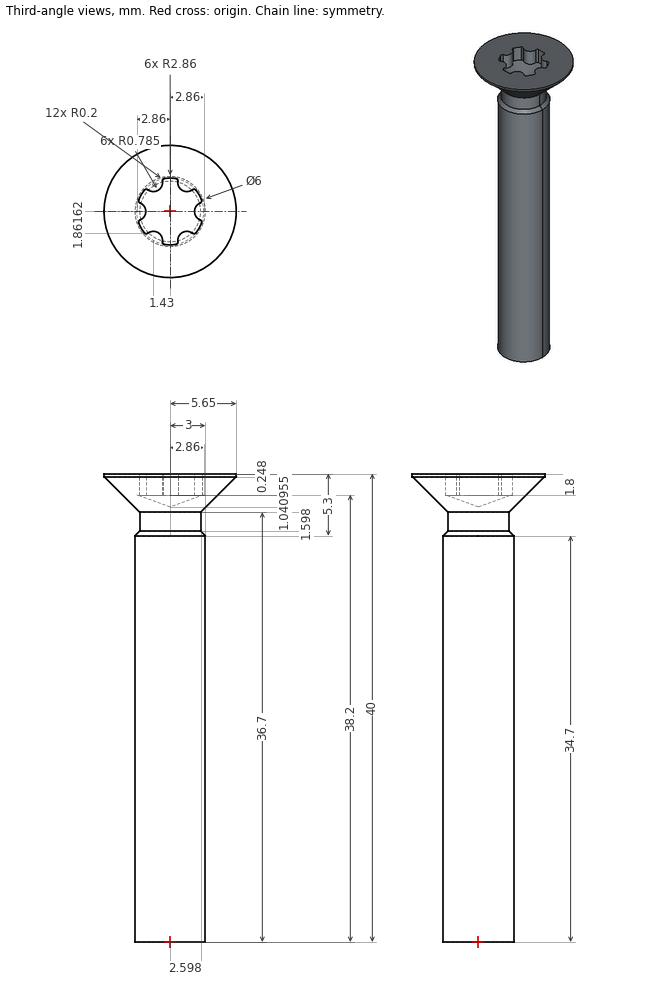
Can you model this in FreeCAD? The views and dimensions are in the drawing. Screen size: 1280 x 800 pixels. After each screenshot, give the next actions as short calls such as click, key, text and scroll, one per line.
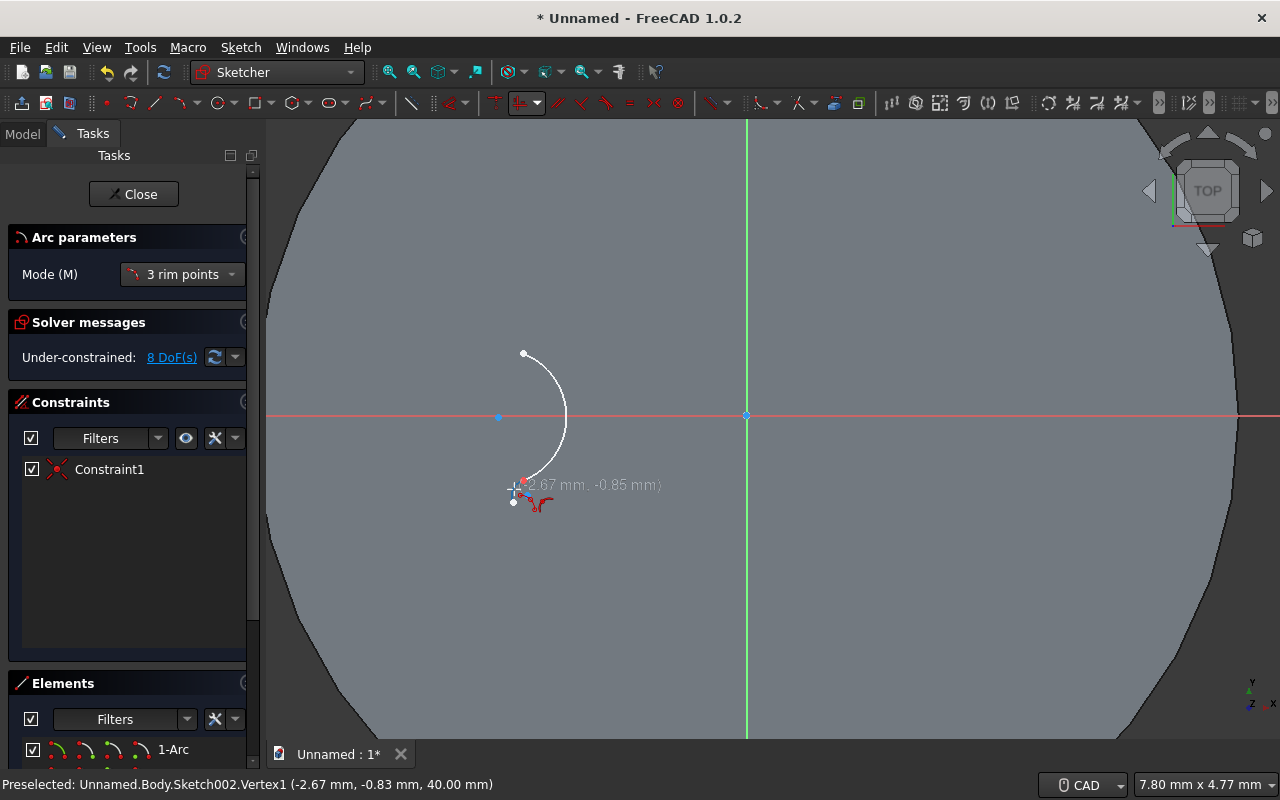
click(514, 500)
click(548, 560)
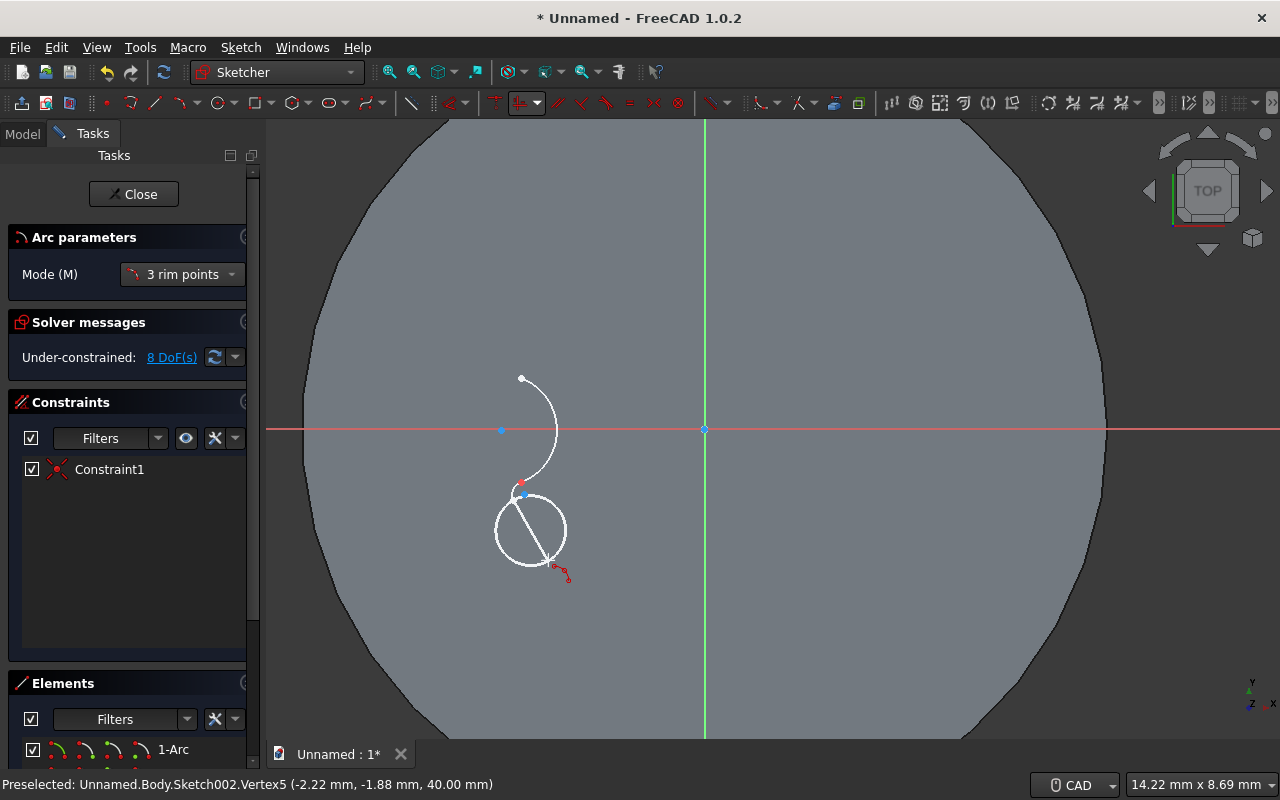
scroll(528, 531, up, 9)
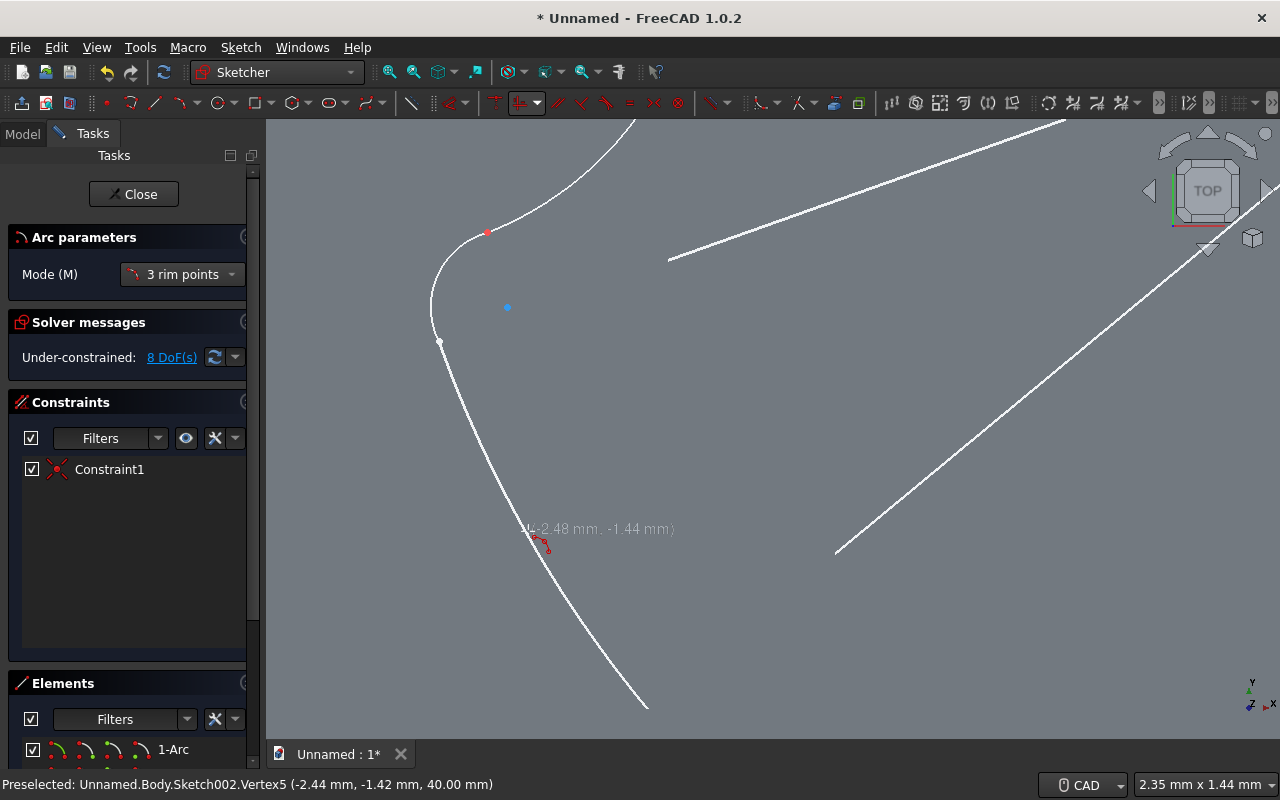
click(526, 529)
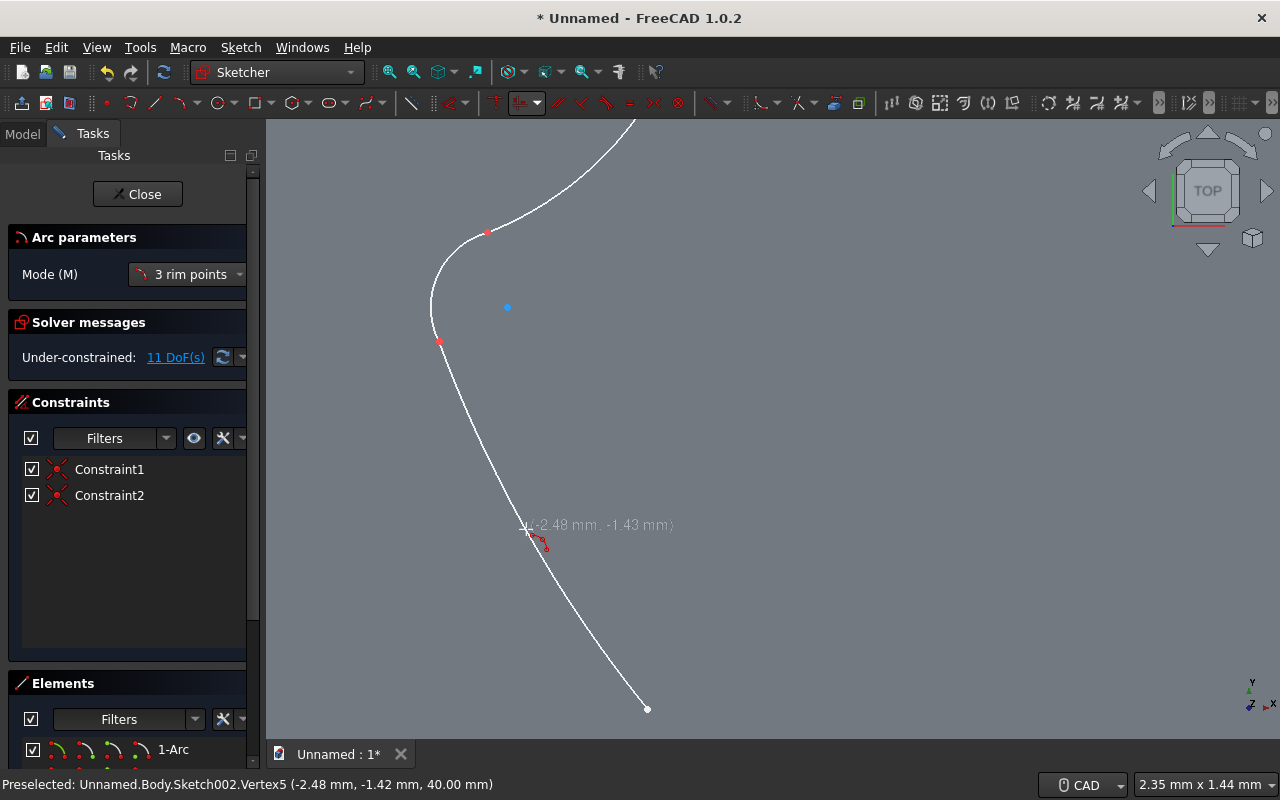
scroll(528, 531, down, 9)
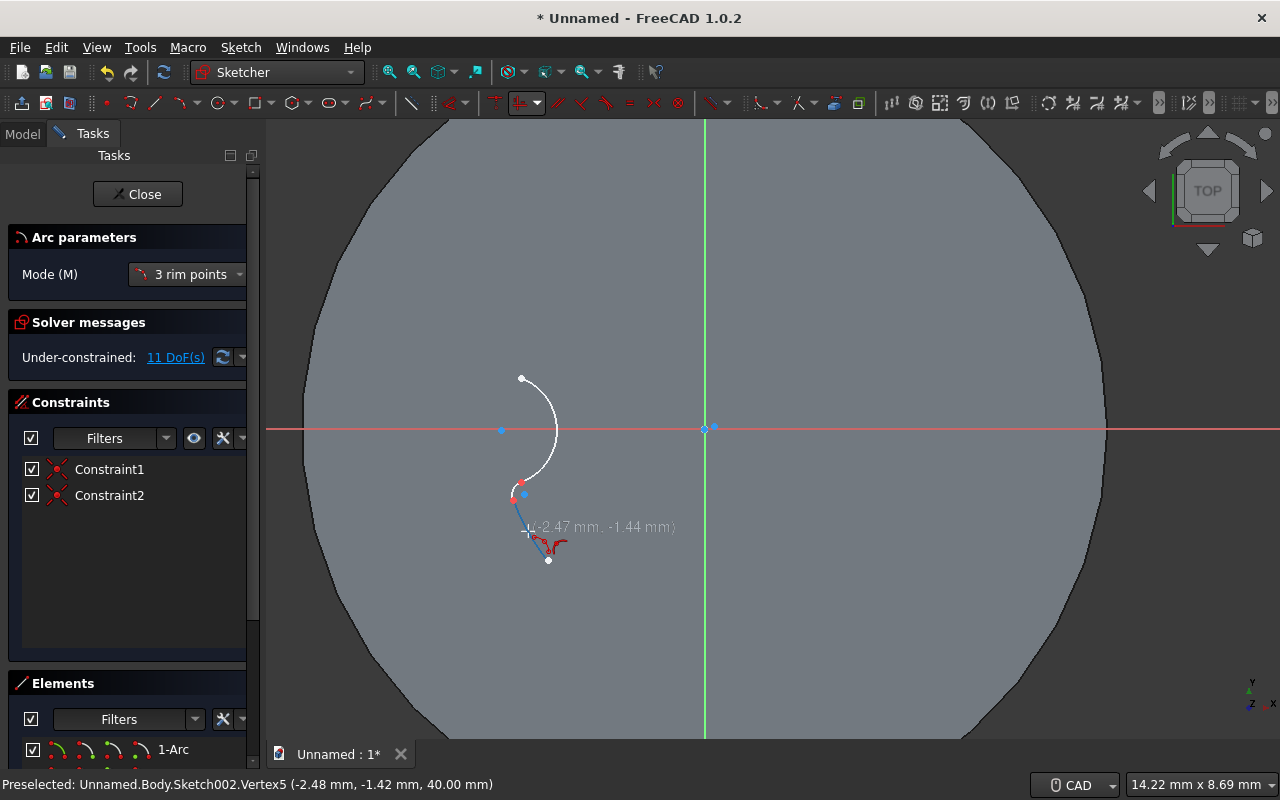
click(548, 561)
click(568, 562)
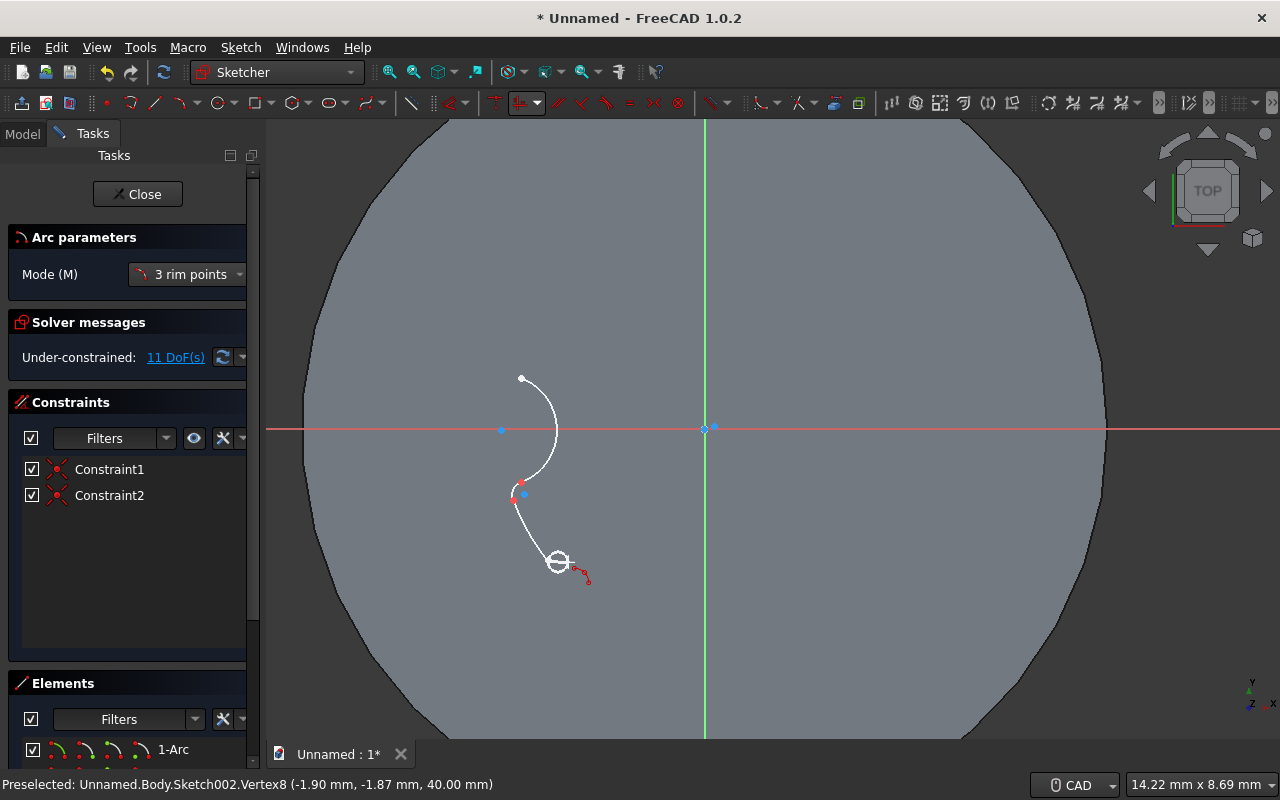
scroll(557, 565, up, 7)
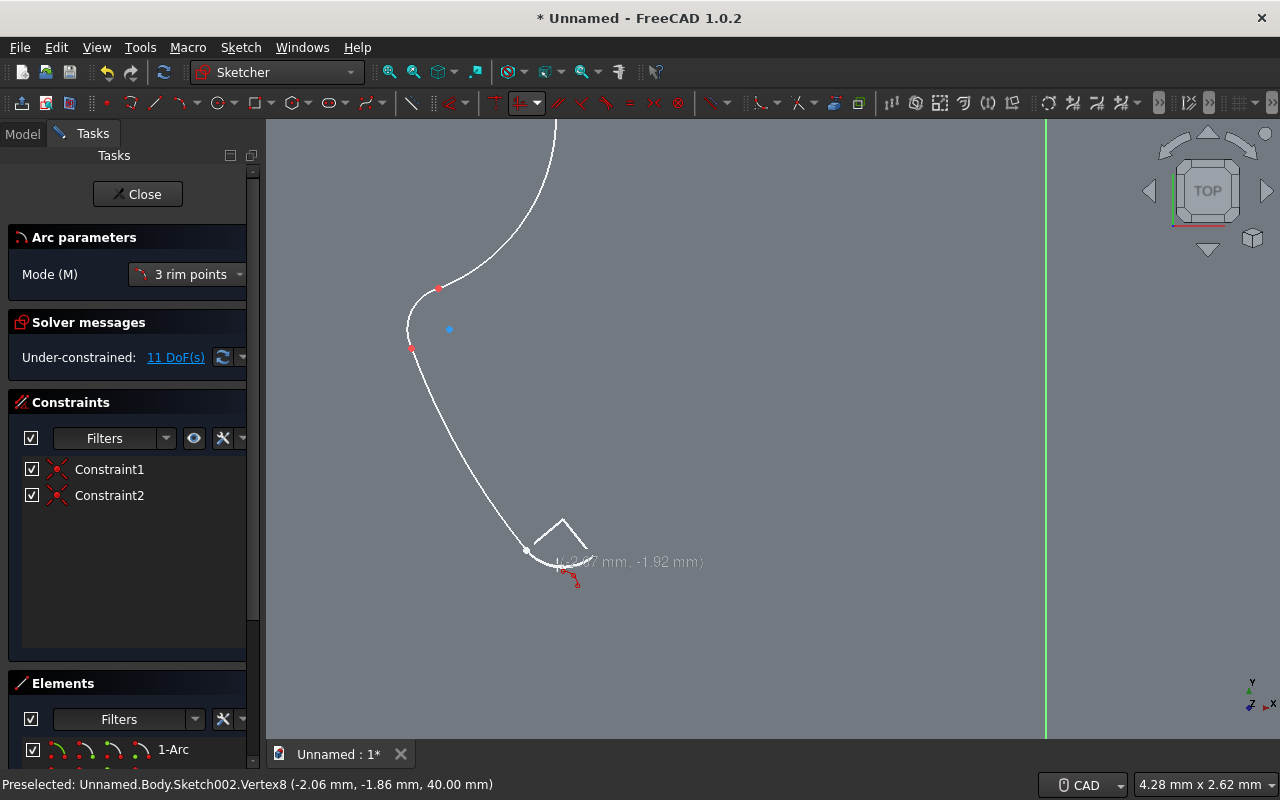
click(558, 563)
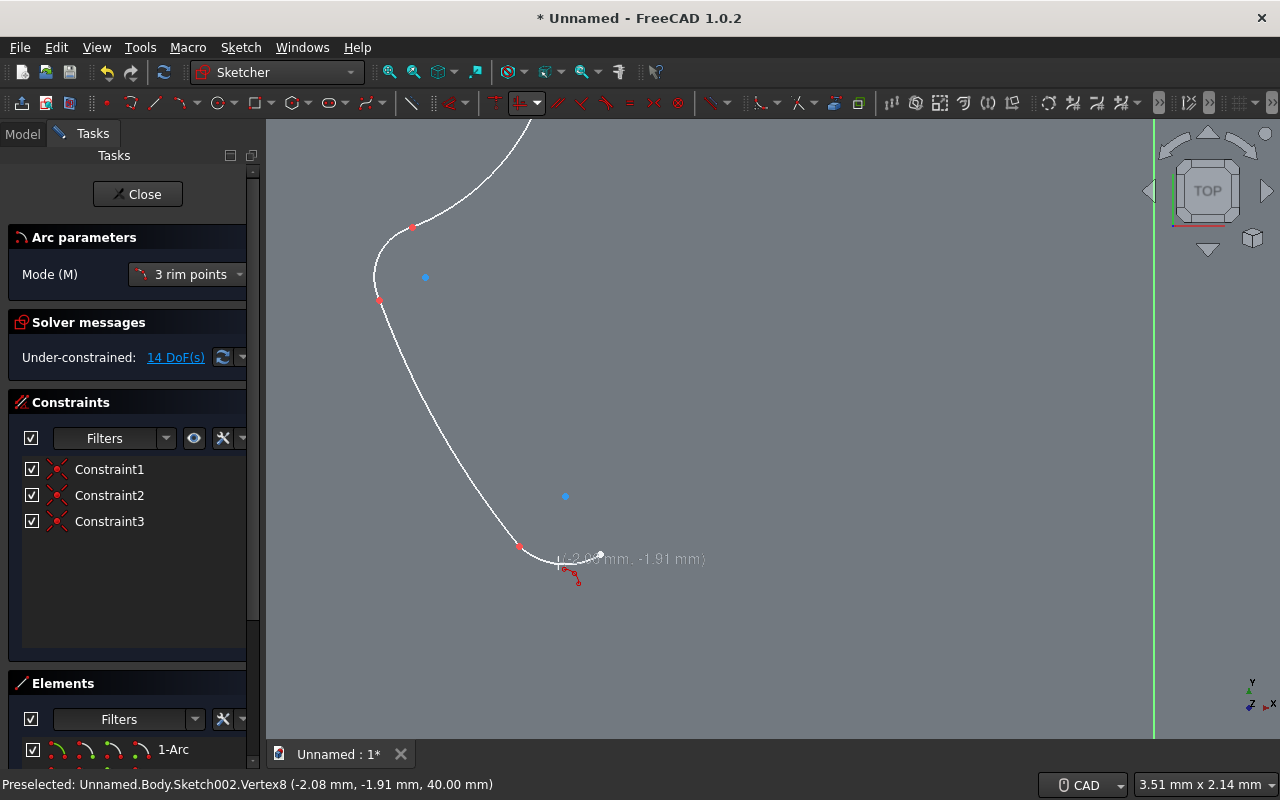
scroll(557, 565, down, 7)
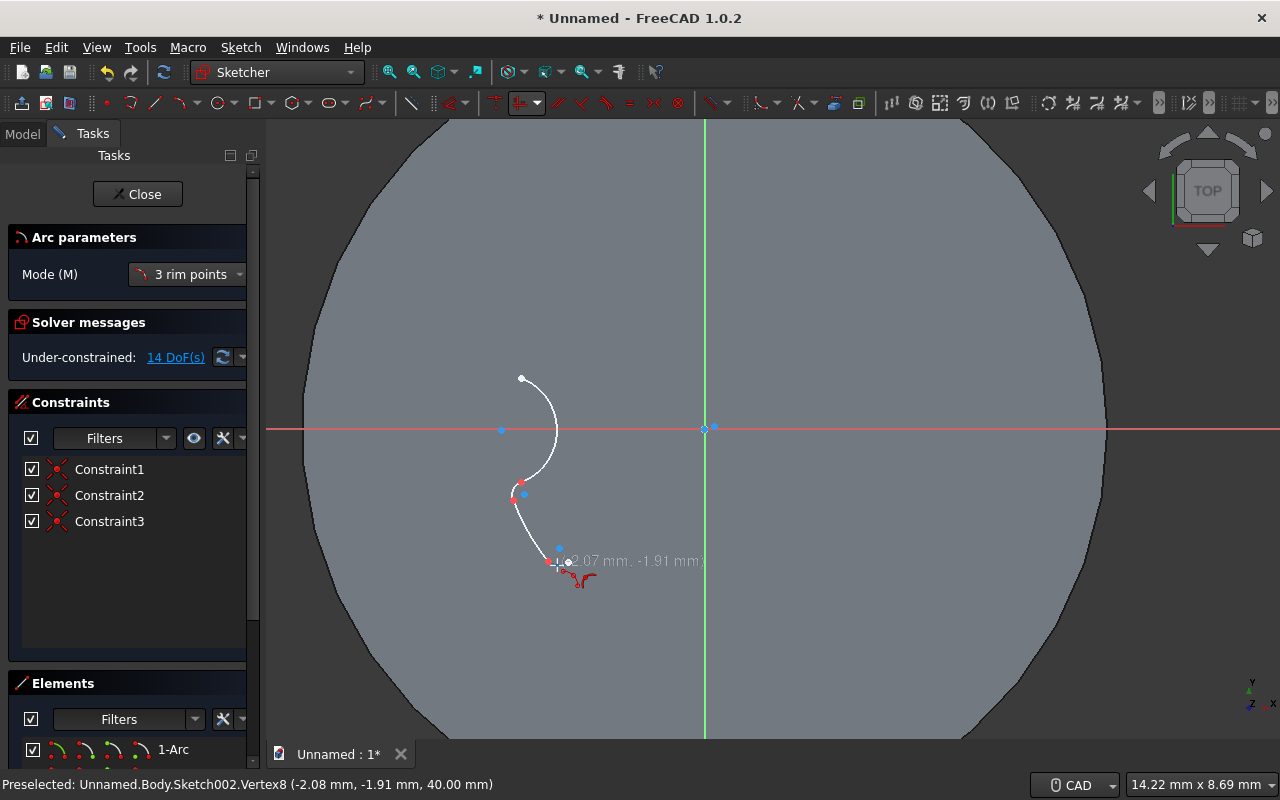
click(568, 563)
click(658, 614)
click(631, 557)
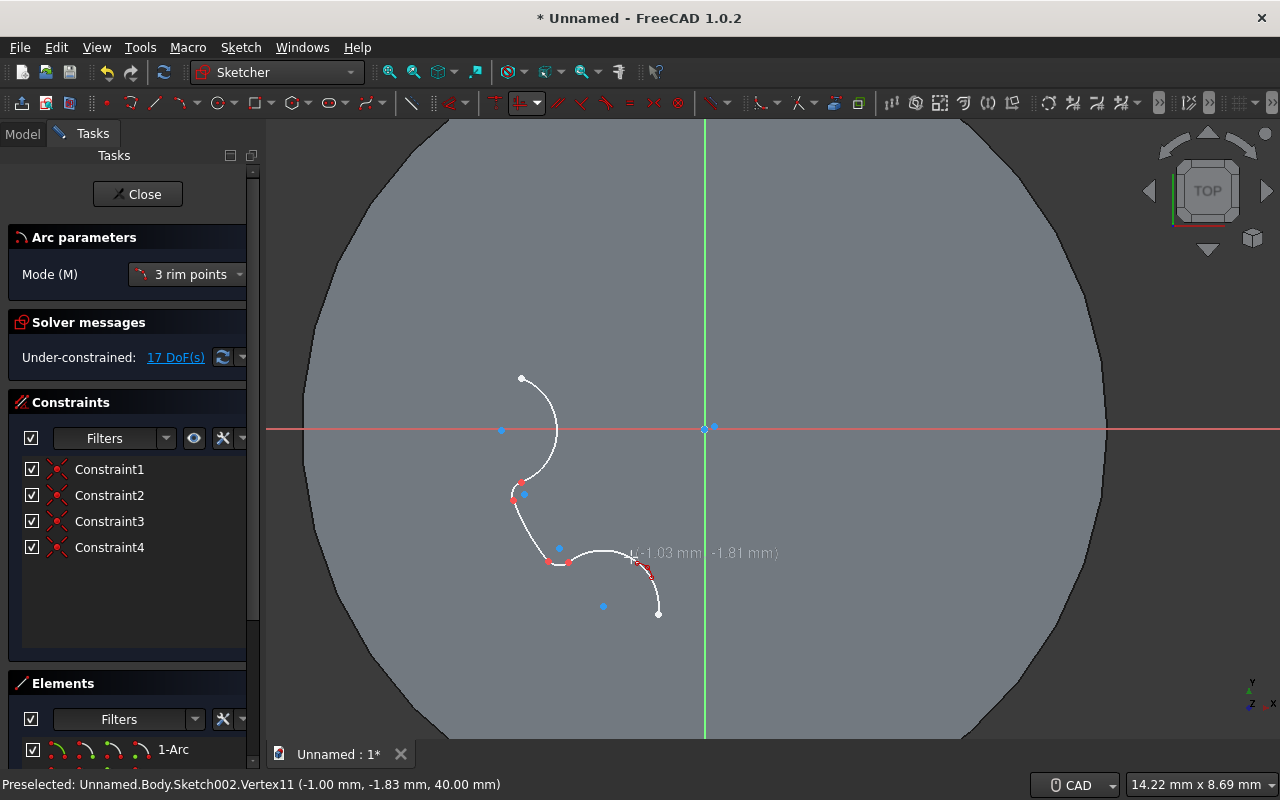
click(658, 615)
click(670, 630)